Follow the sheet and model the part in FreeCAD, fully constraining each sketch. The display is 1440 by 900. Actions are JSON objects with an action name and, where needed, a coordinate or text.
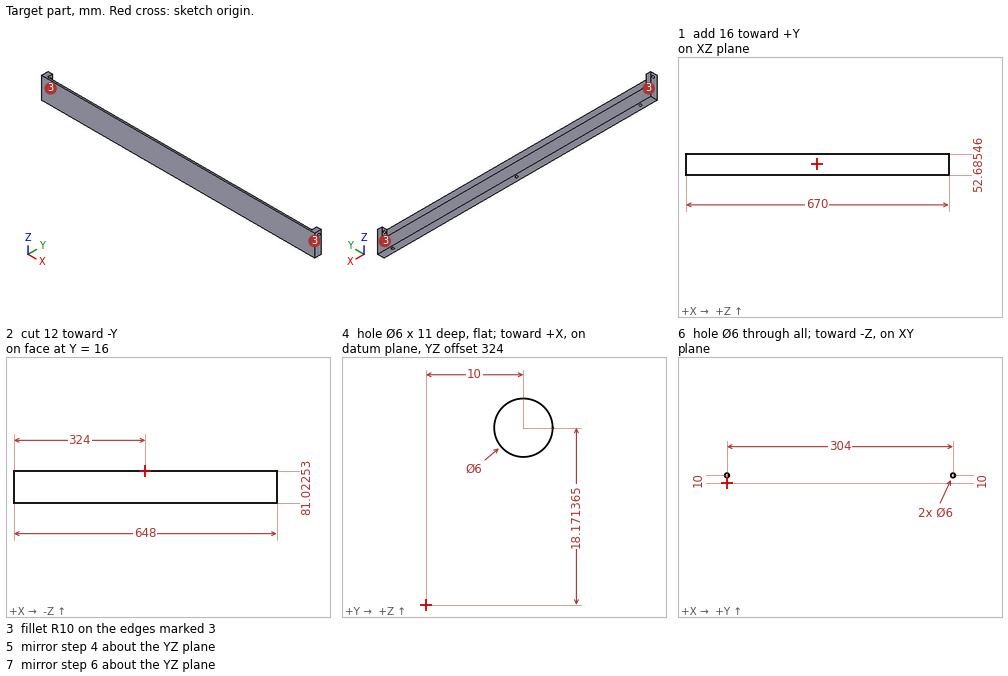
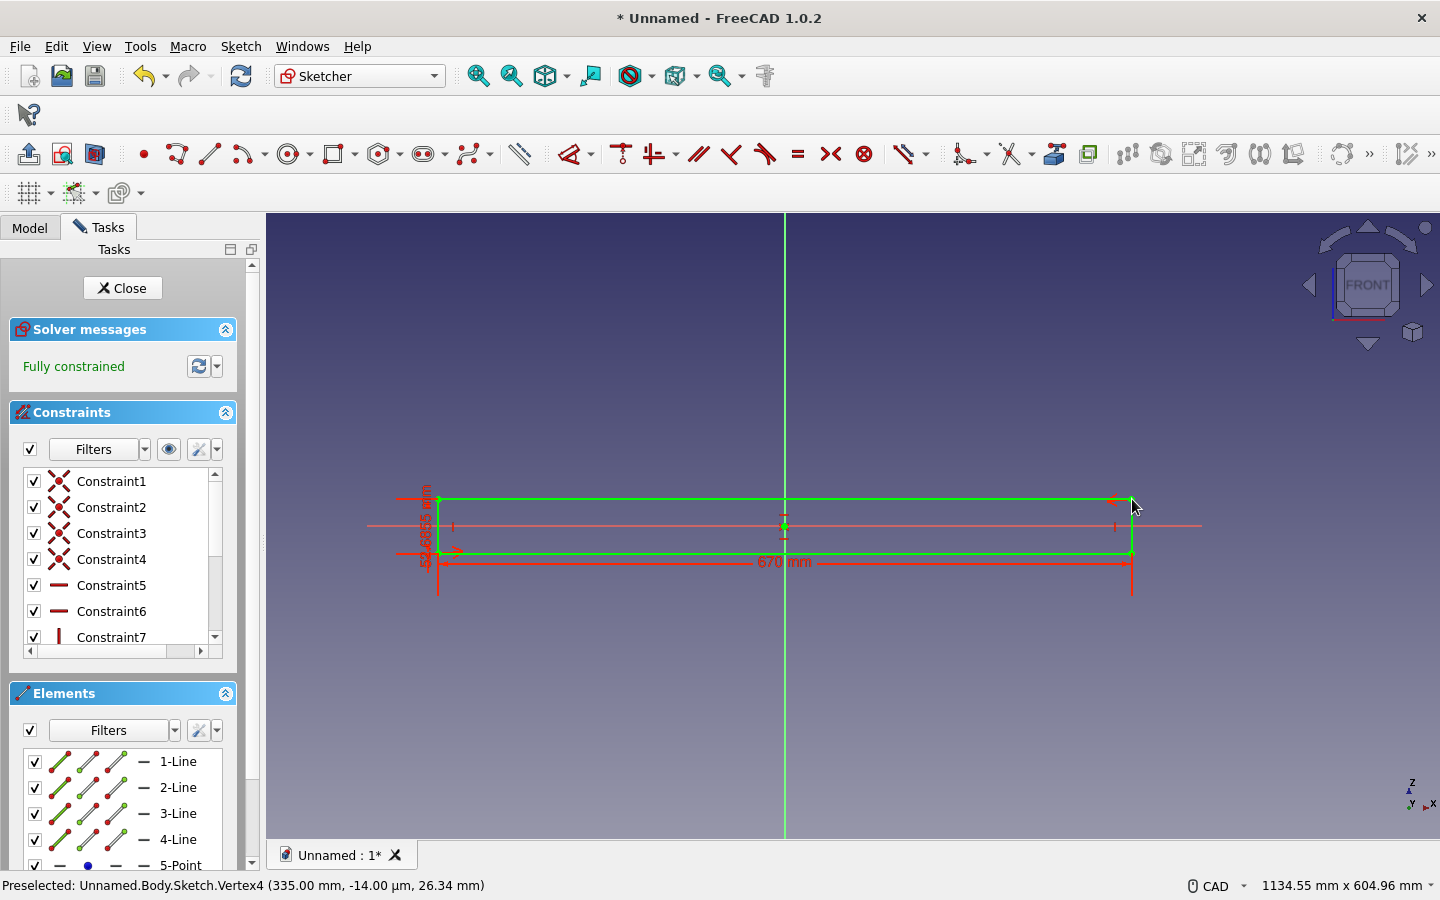
{"action": "left_click", "coordinate": [123, 288]}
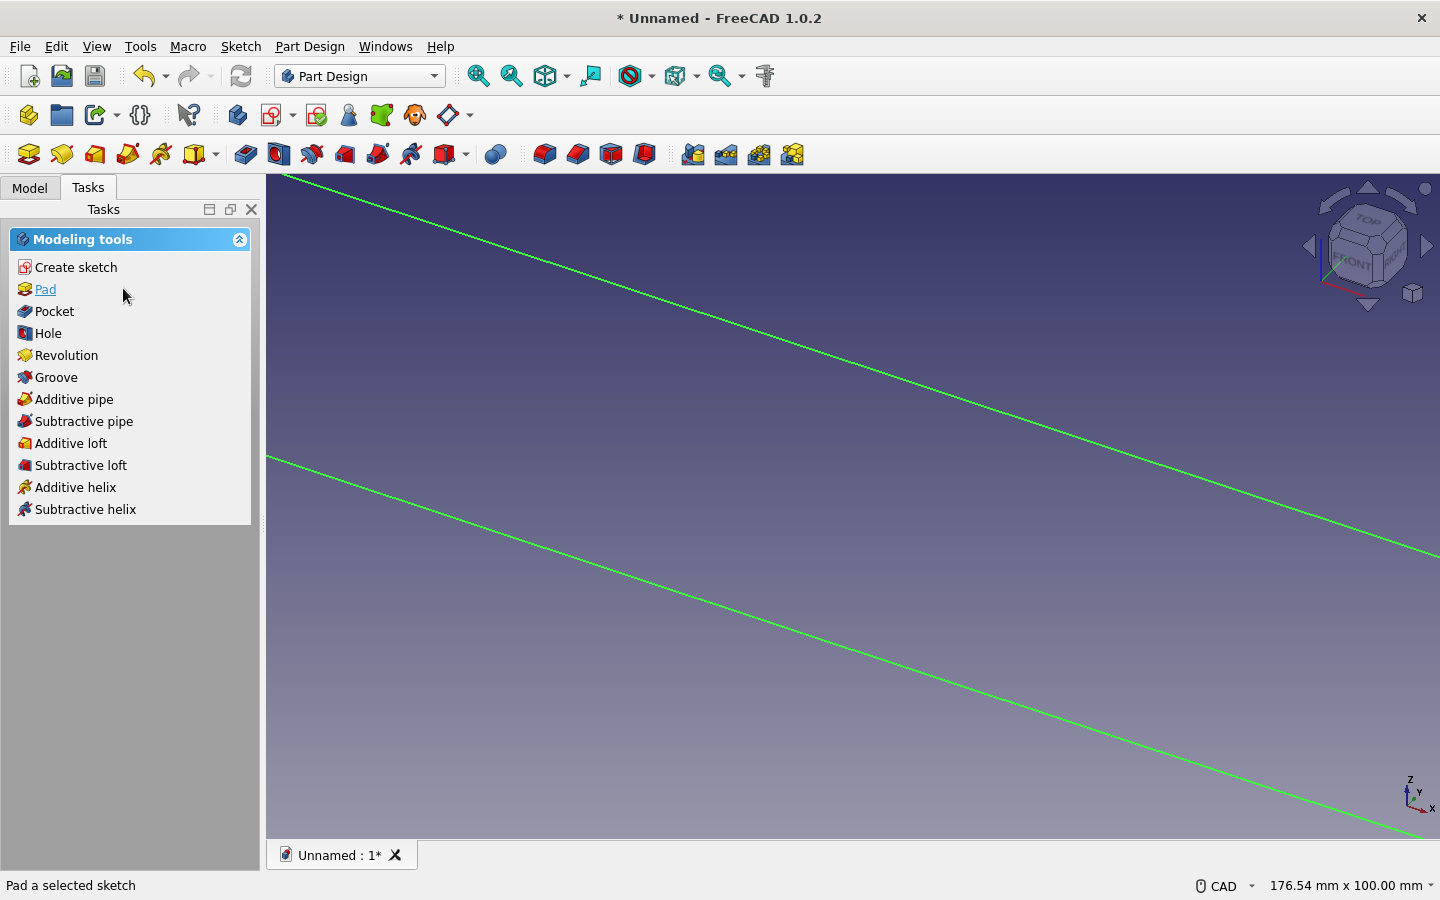
{"action": "left_click", "coordinate": [29, 154]}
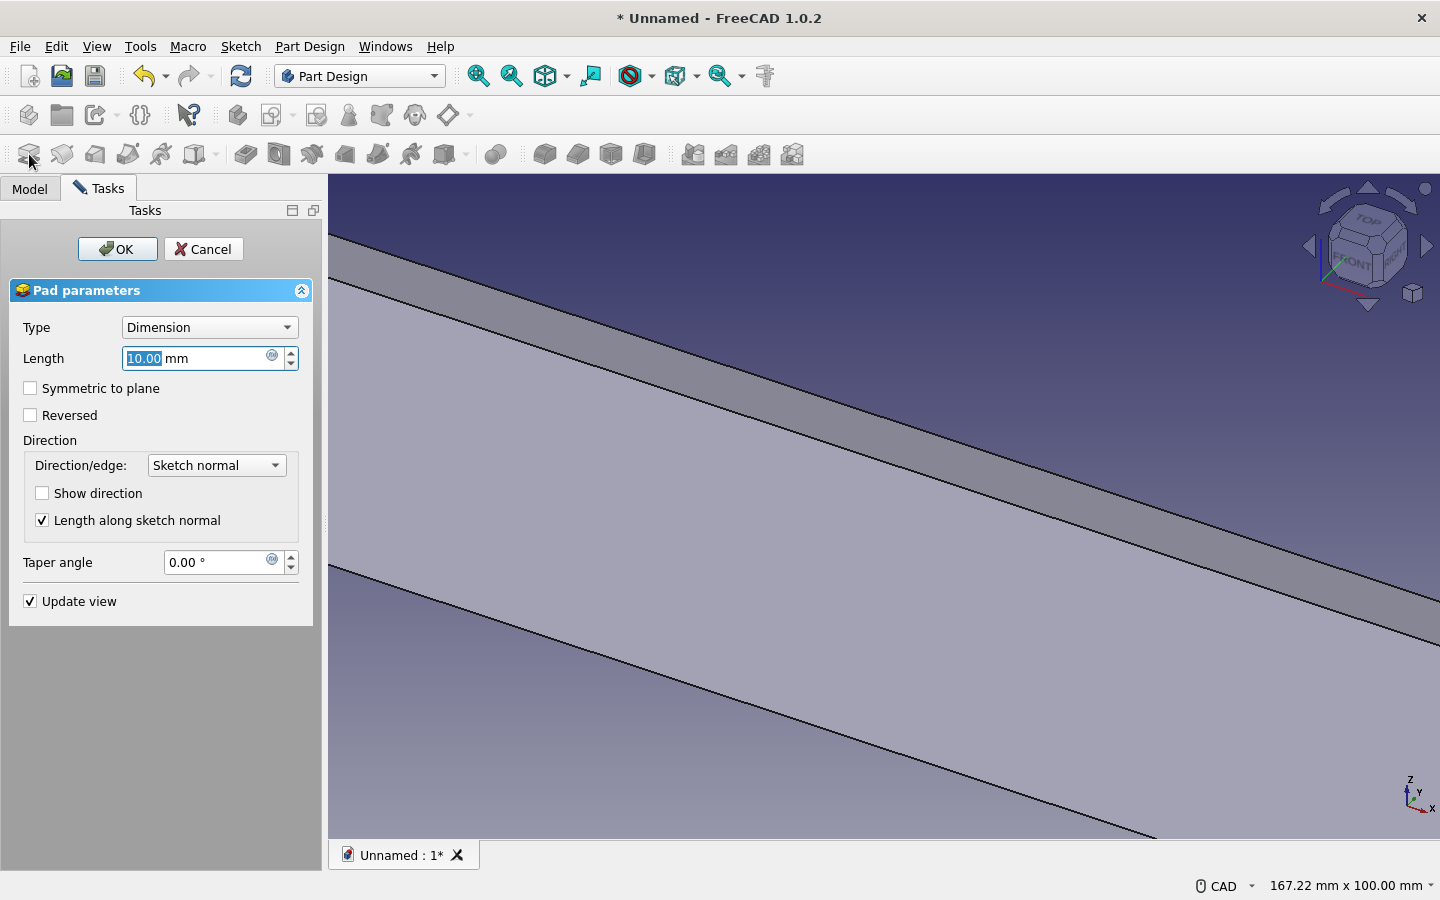
{"action": "type", "text": "16"}
{"action": "key", "text": "Tab"}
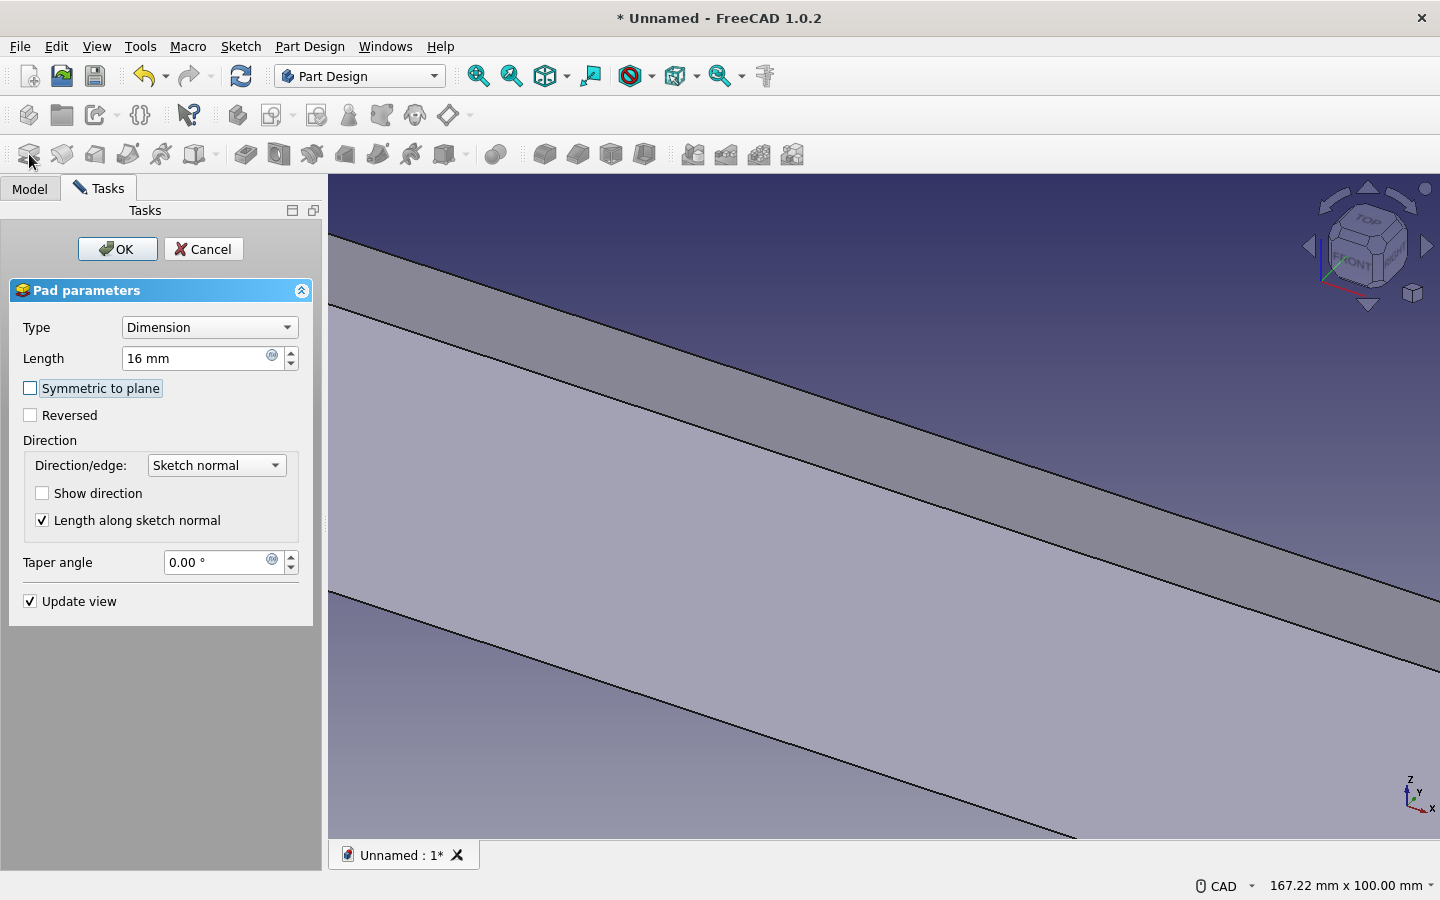
{"action": "left_click", "coordinate": [31, 415]}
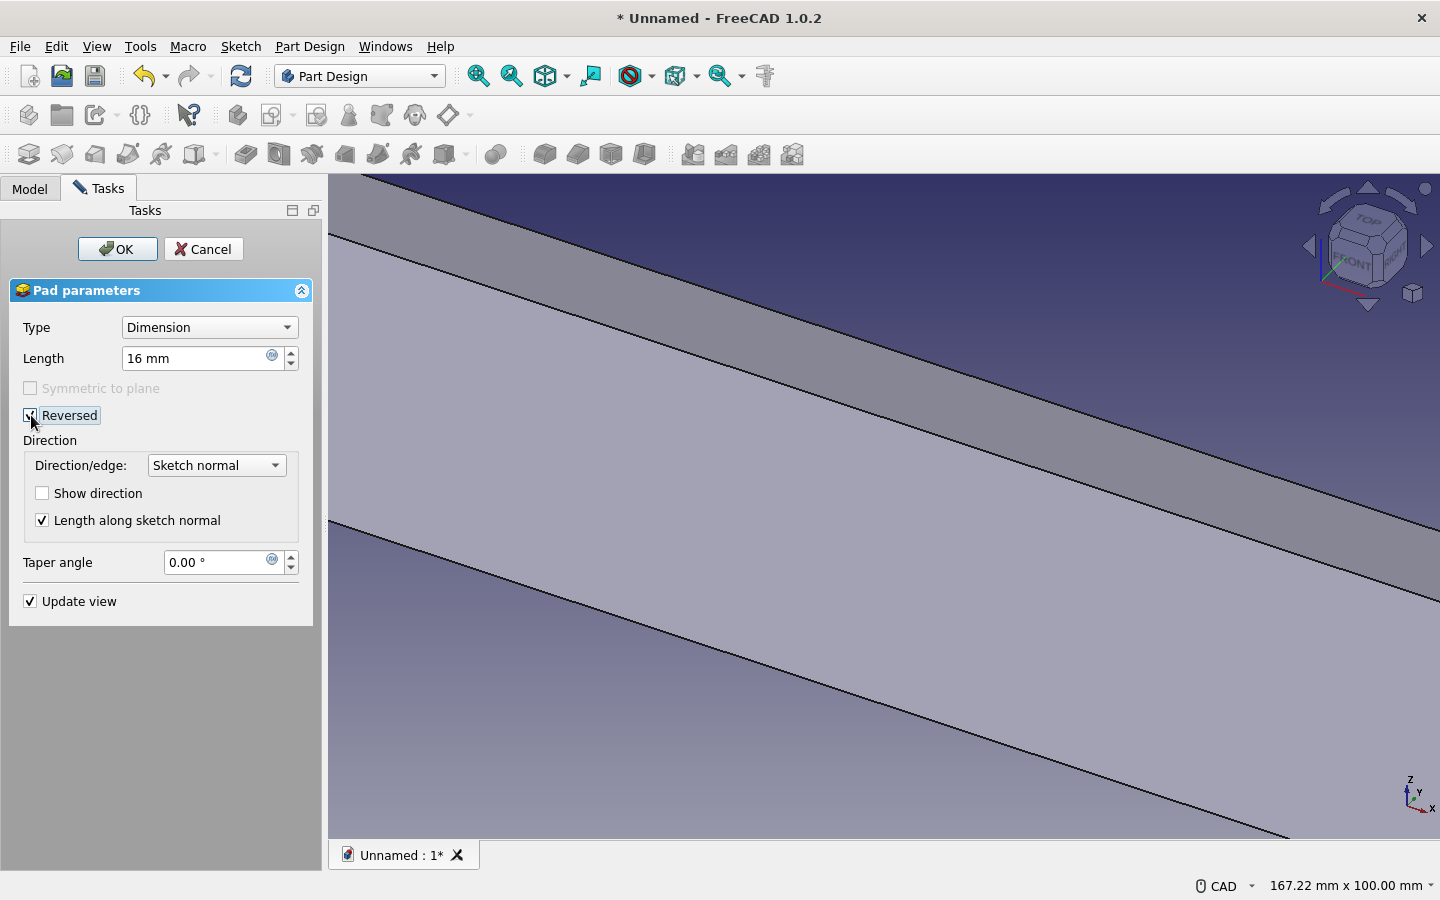
{"action": "left_click", "coordinate": [118, 249]}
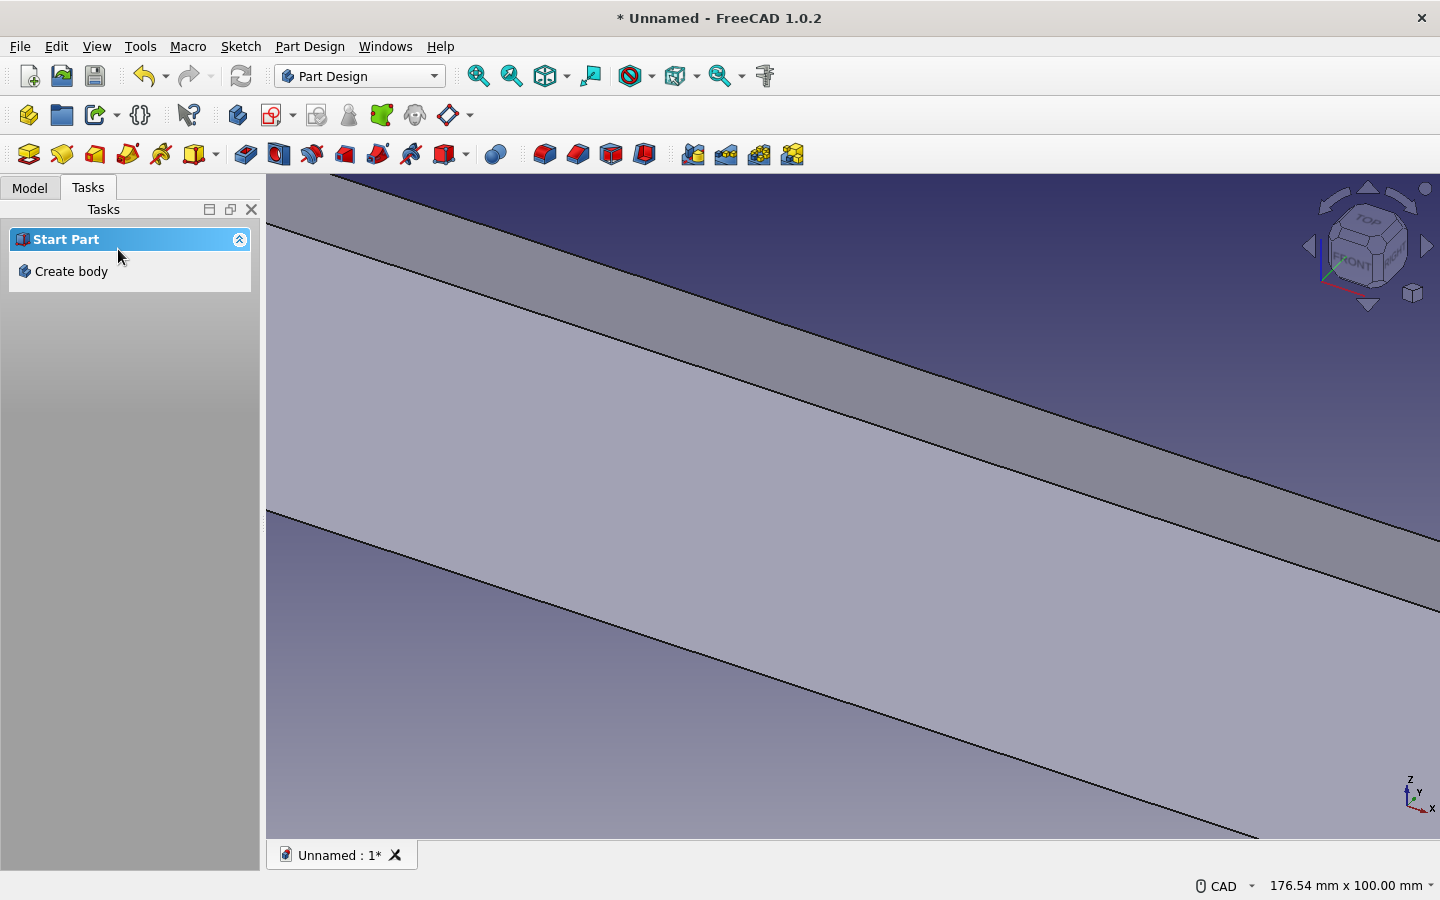
{"action": "left_click", "coordinate": [479, 76]}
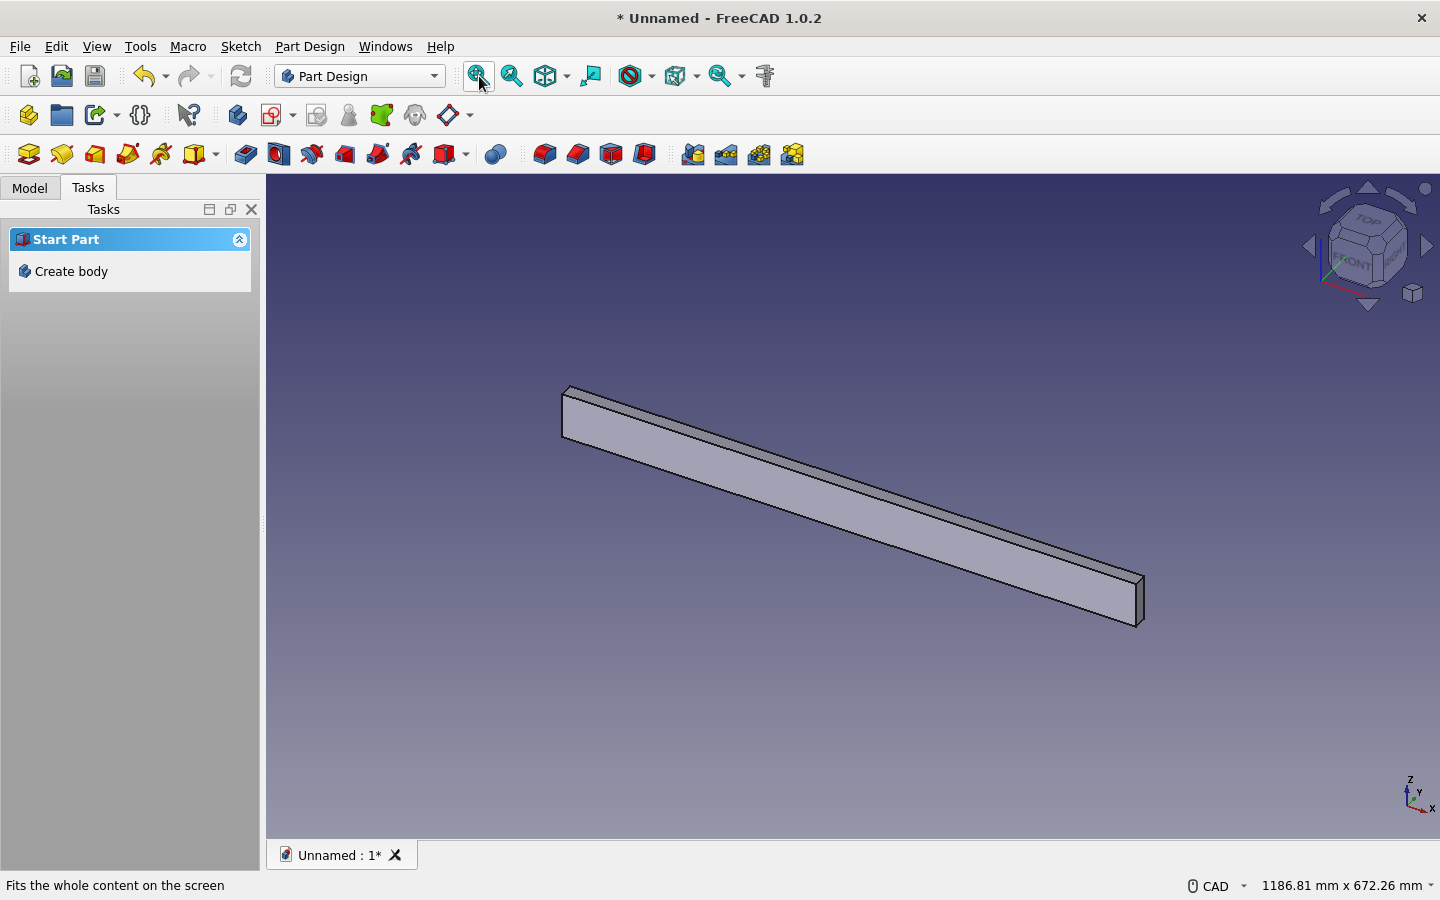
{"action": "key", "text": "4"}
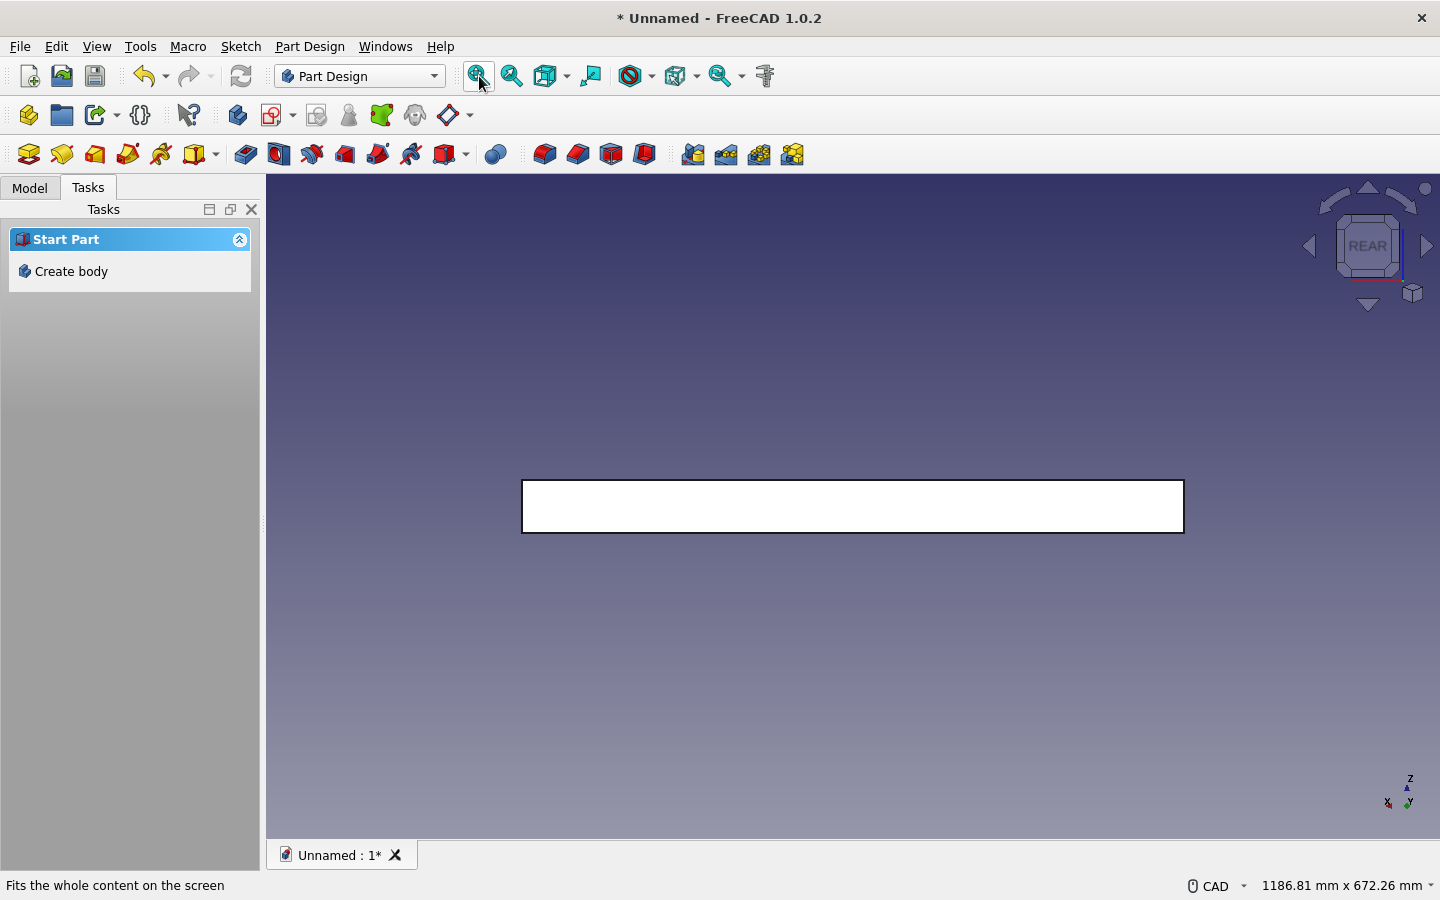
{"action": "left_click", "coordinate": [569, 506]}